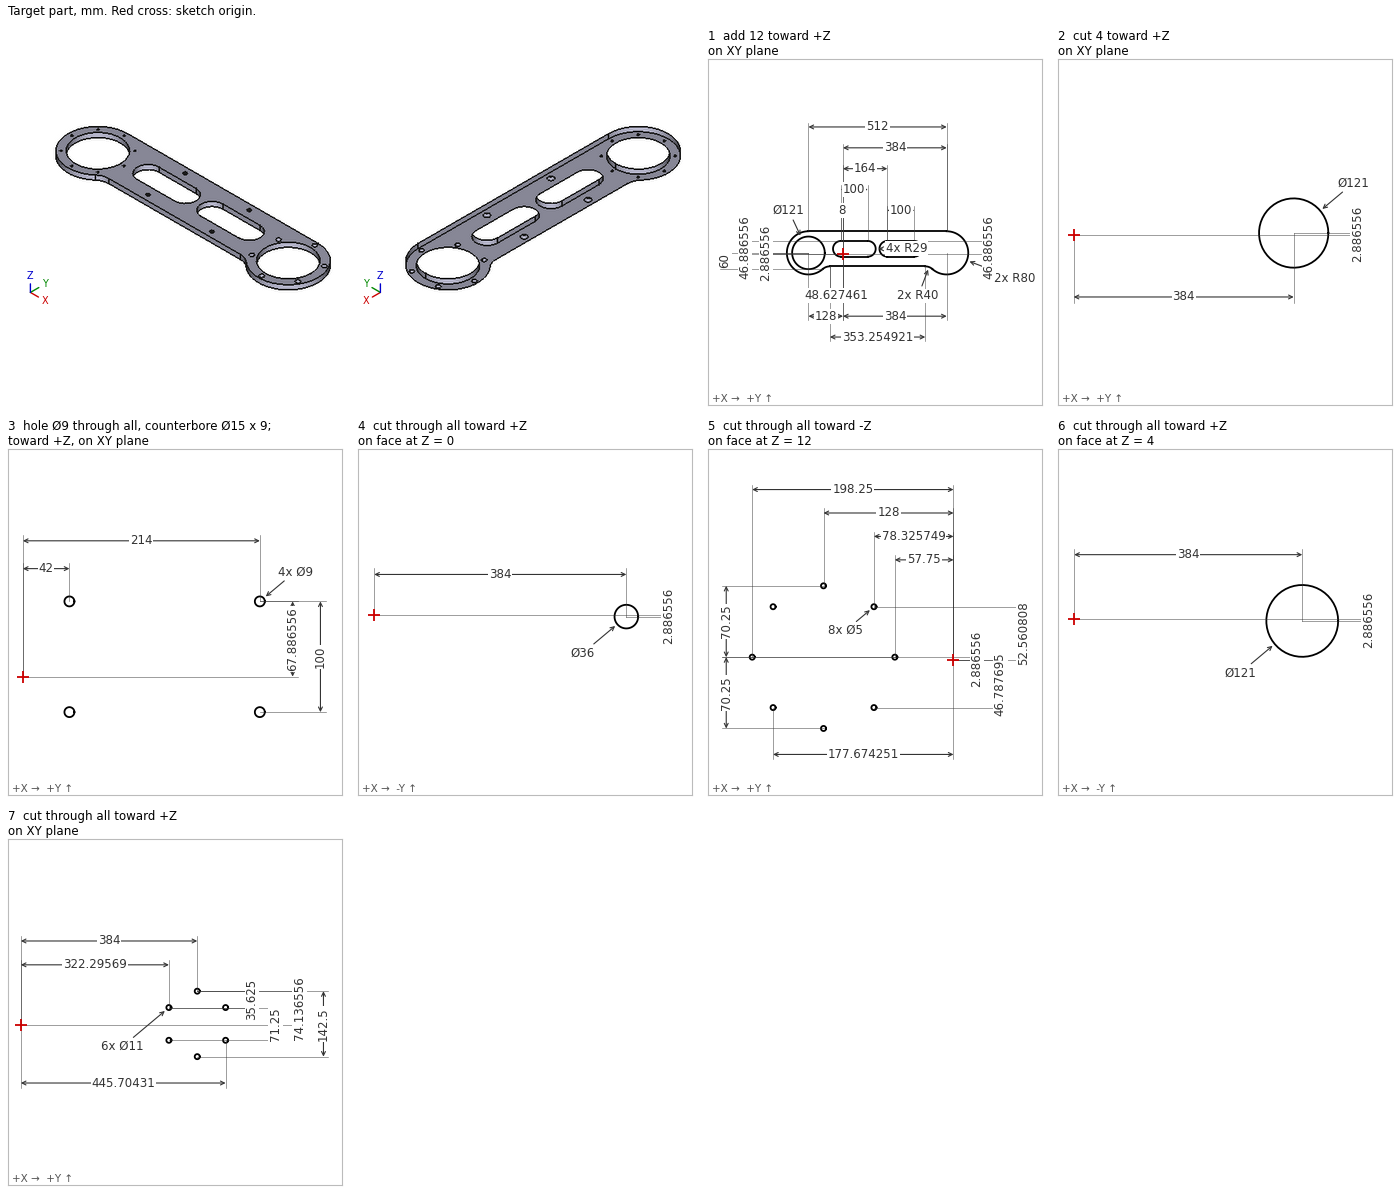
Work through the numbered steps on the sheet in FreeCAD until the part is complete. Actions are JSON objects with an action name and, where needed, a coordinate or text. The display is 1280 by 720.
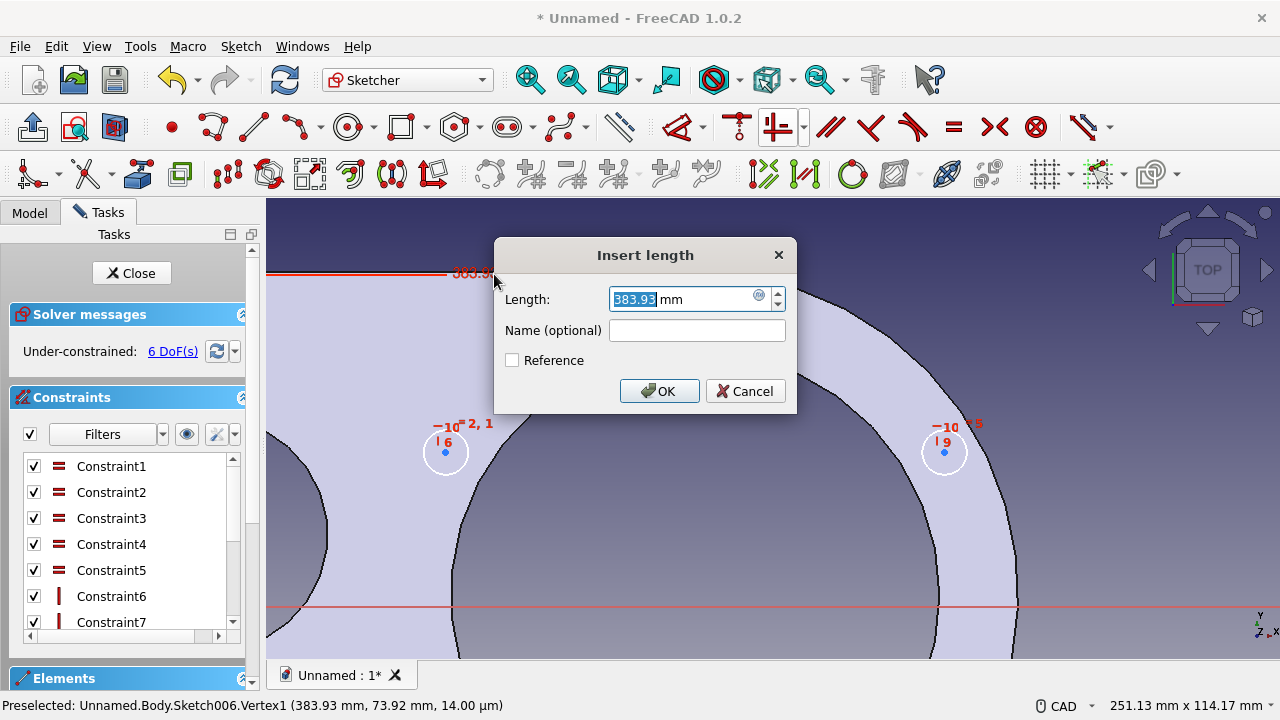
{"action": "type", "text": "384"}
{"action": "key", "text": "Return"}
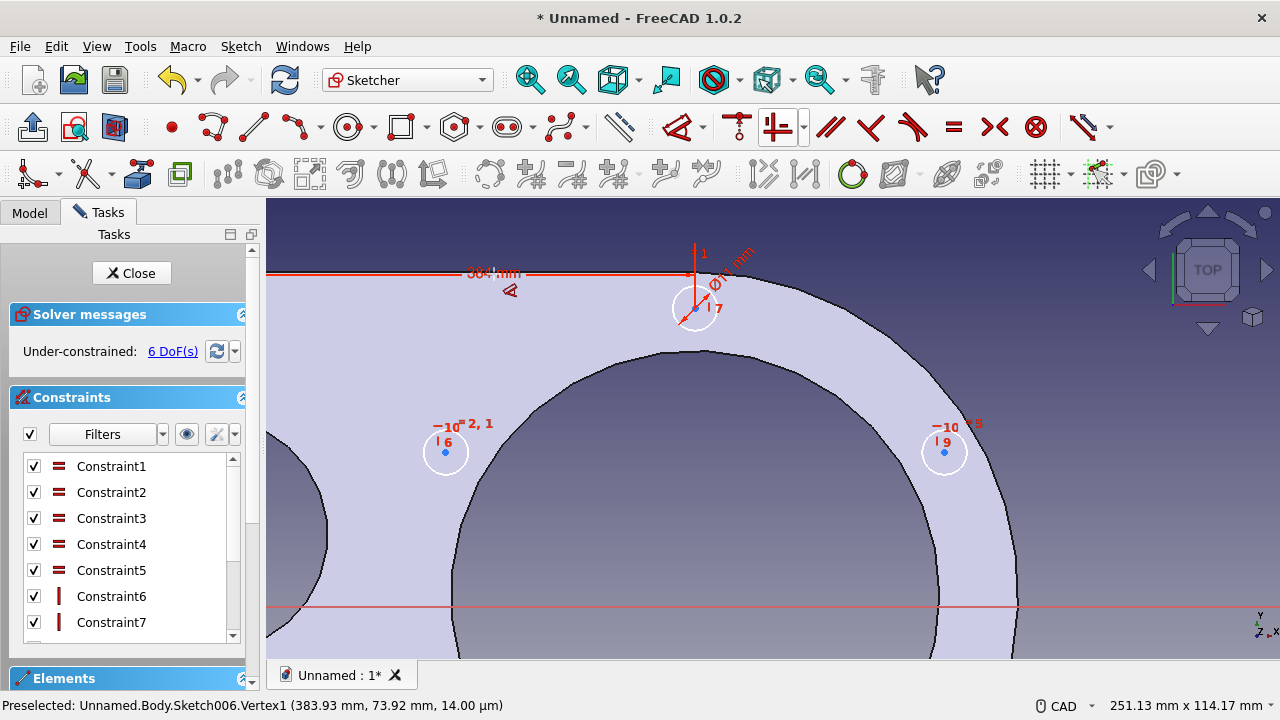
{"action": "left_click", "coordinate": [446, 453]}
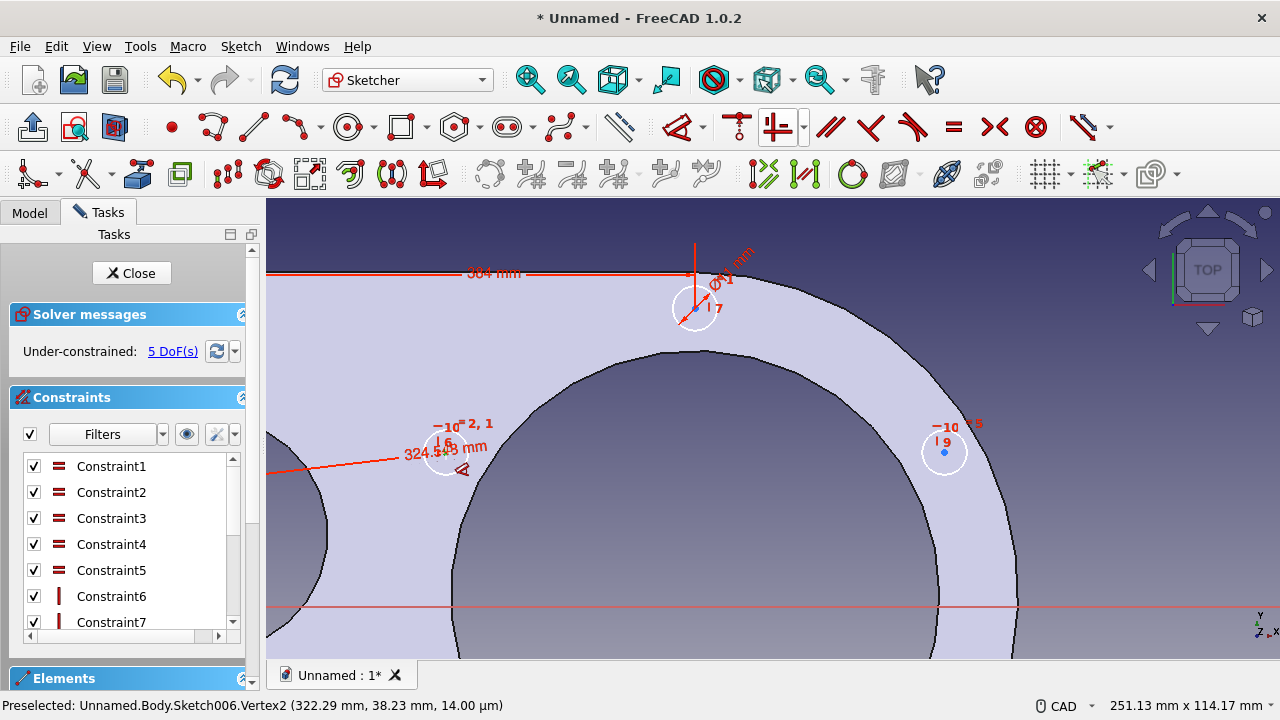
{"action": "scroll", "coordinate": [712, 292], "scroll_direction": "down", "scroll_amount": 4}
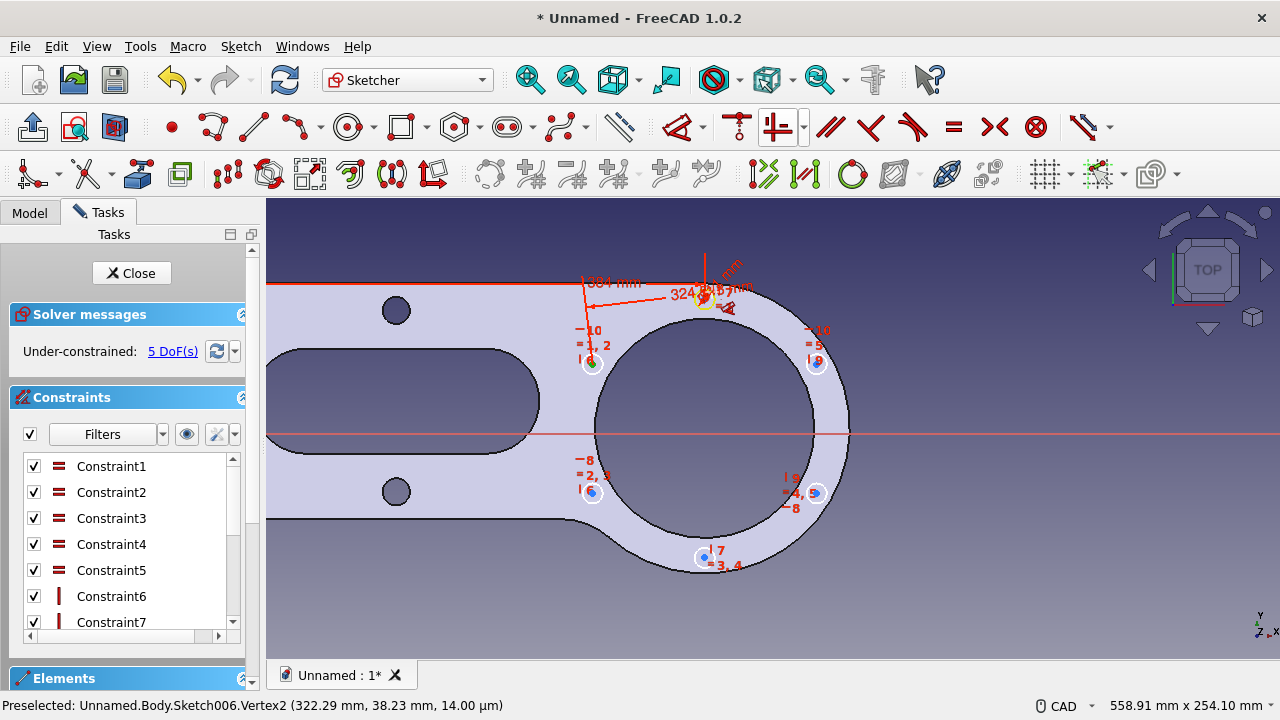
{"action": "left_click", "coordinate": [593, 493]}
{"action": "left_click", "coordinate": [559, 399]}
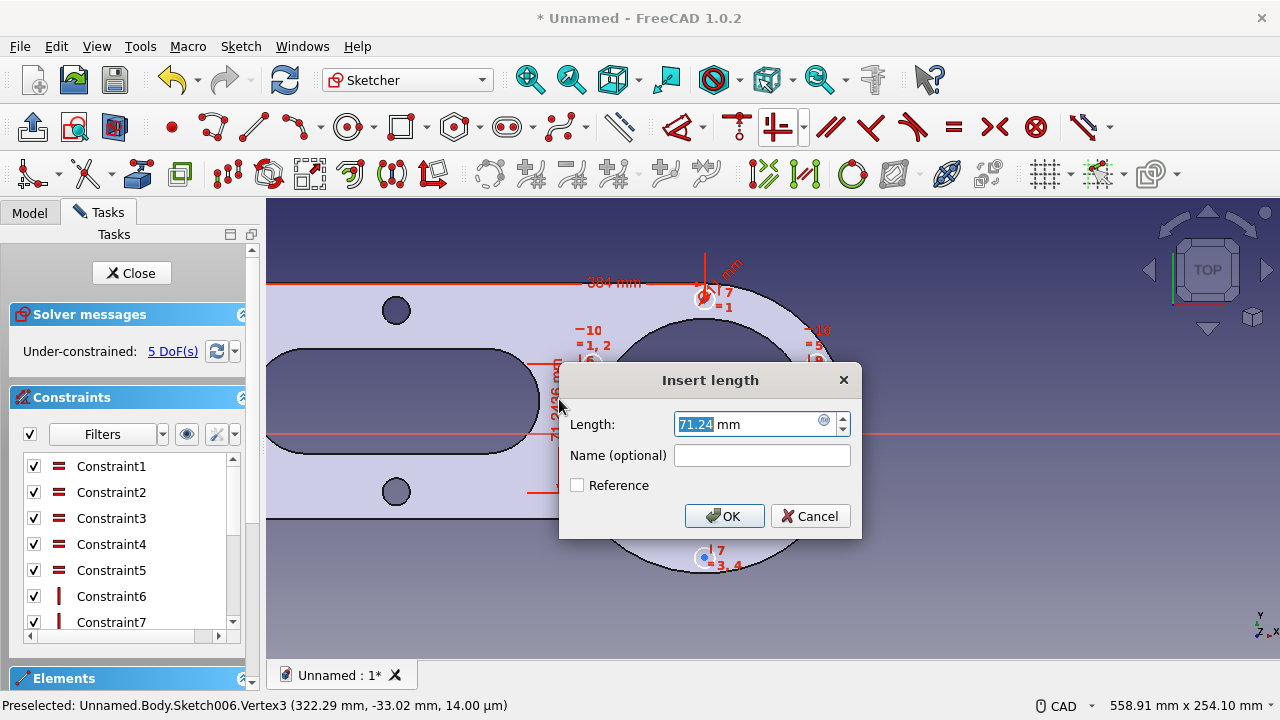
{"action": "type", "text": "71.25"}
{"action": "key", "text": "Return"}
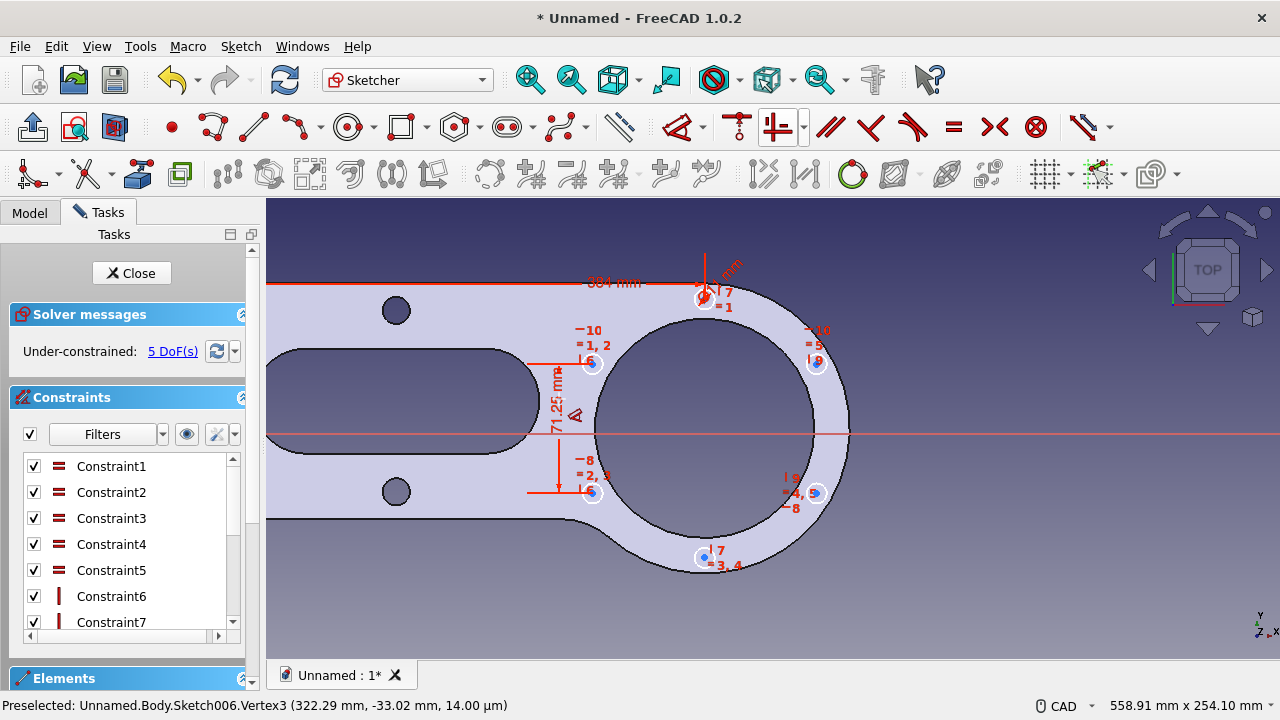
{"action": "left_click", "coordinate": [705, 299]}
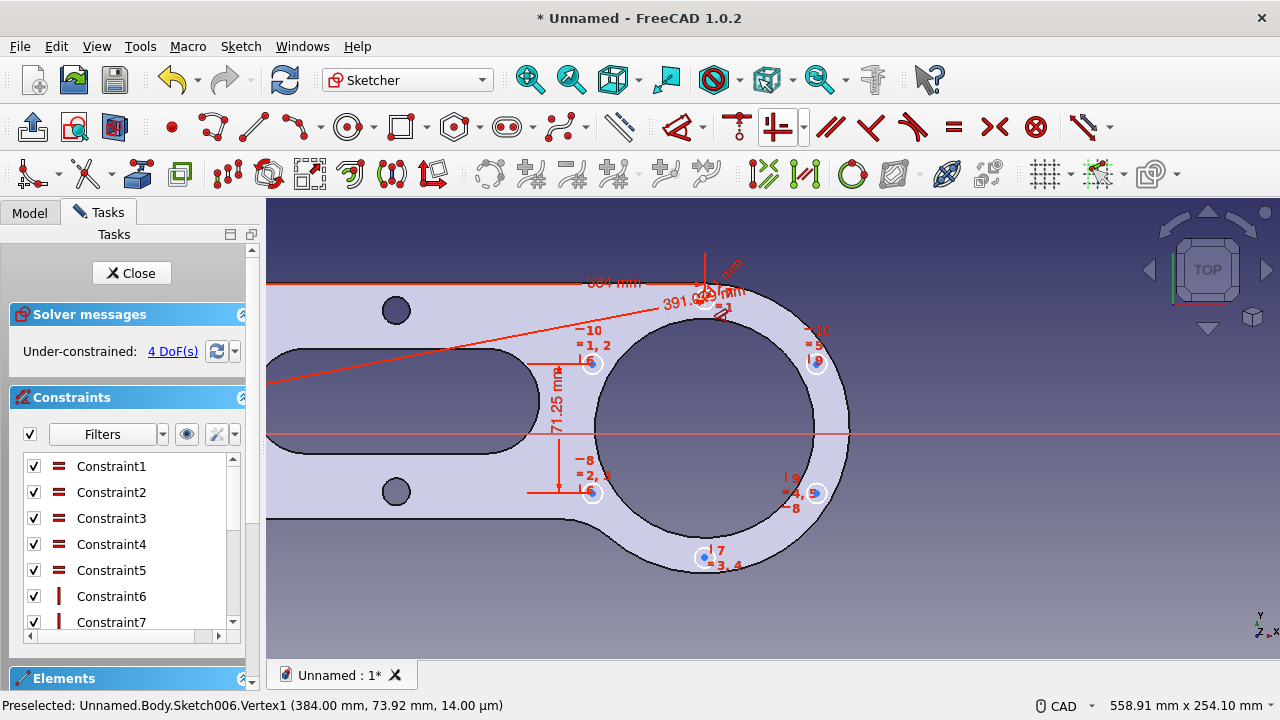
{"action": "left_click", "coordinate": [705, 558]}
{"action": "left_click", "coordinate": [739, 369]}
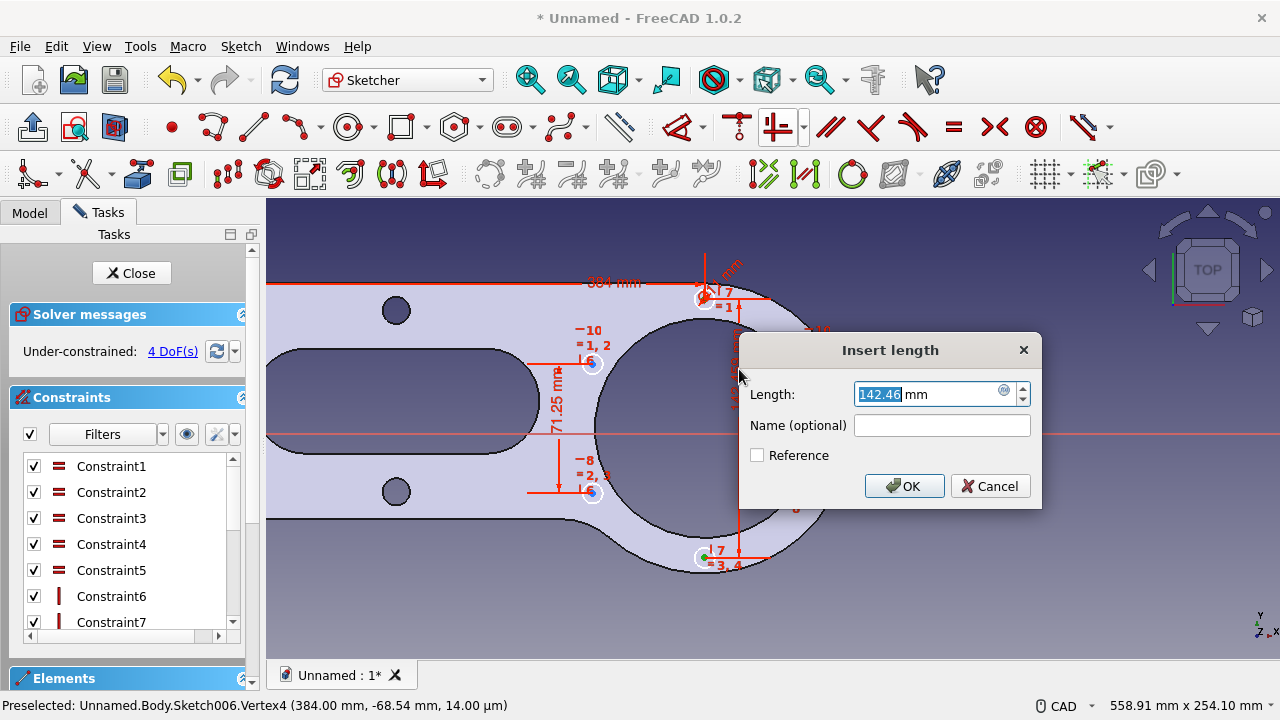
{"action": "type", "text": "142.5"}
{"action": "key", "text": "Return"}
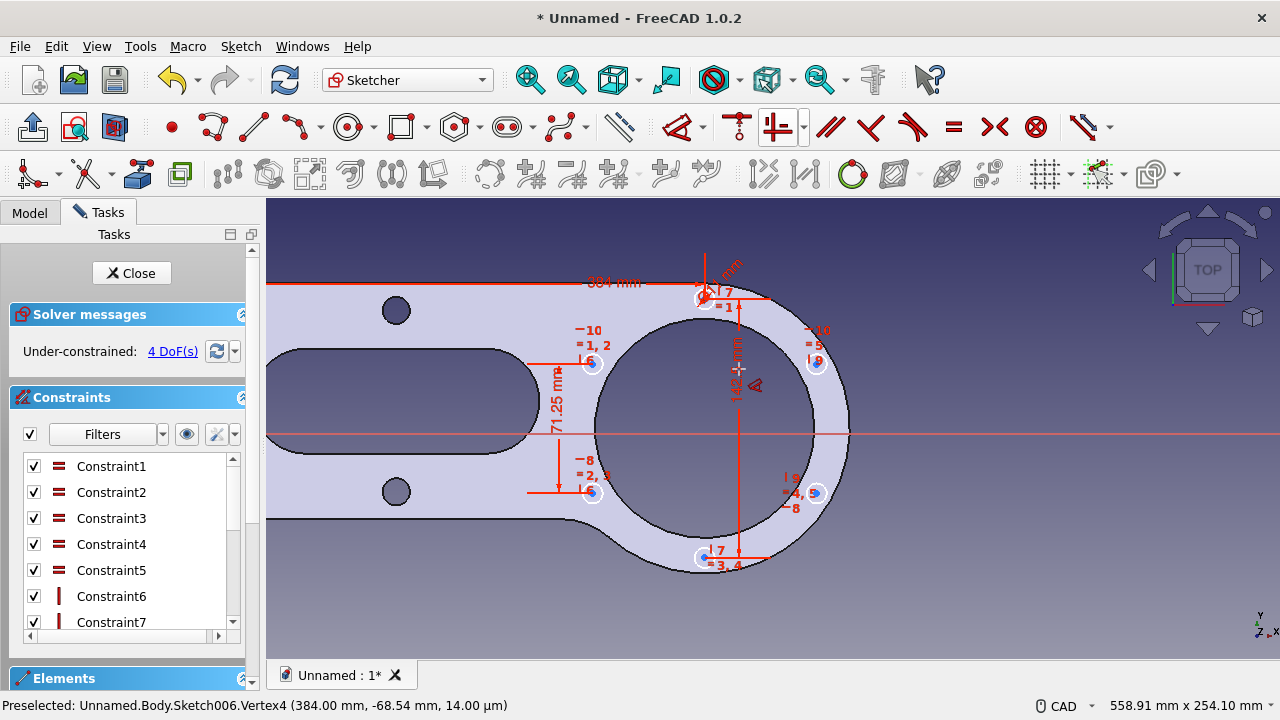
{"action": "left_click", "coordinate": [705, 299]}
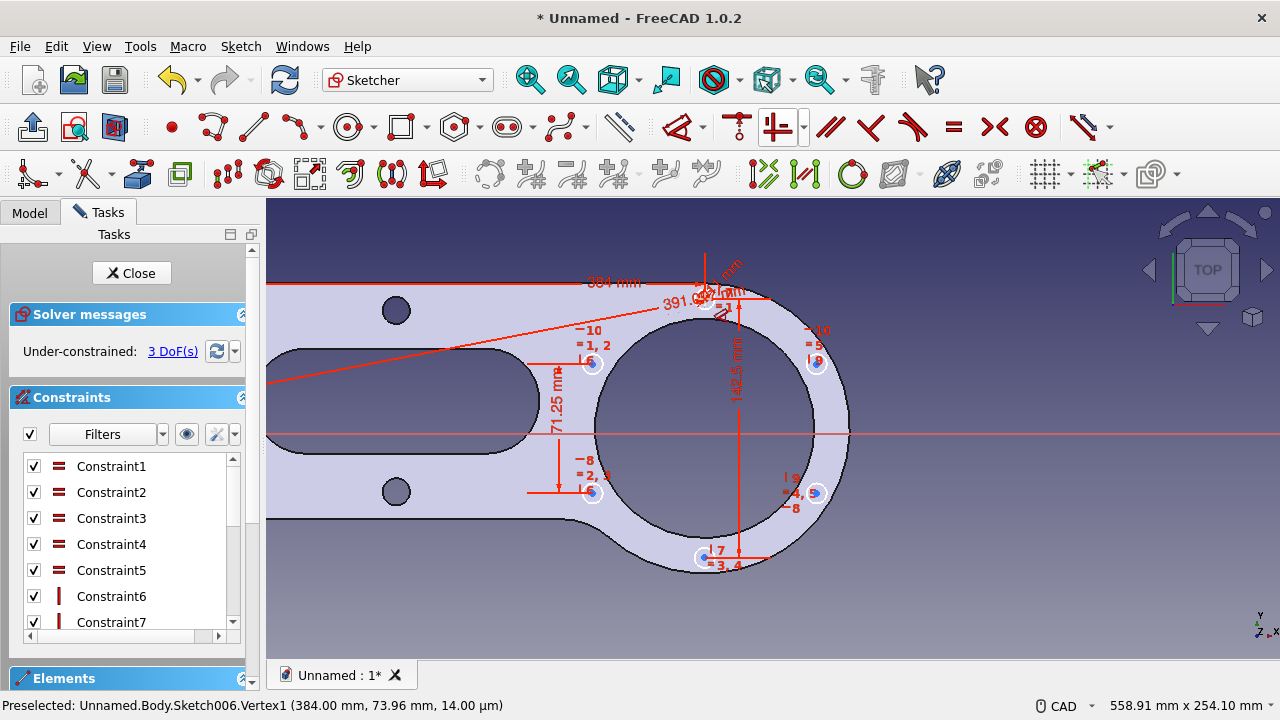
{"action": "left_click", "coordinate": [593, 364]}
{"action": "left_click", "coordinate": [559, 332]}